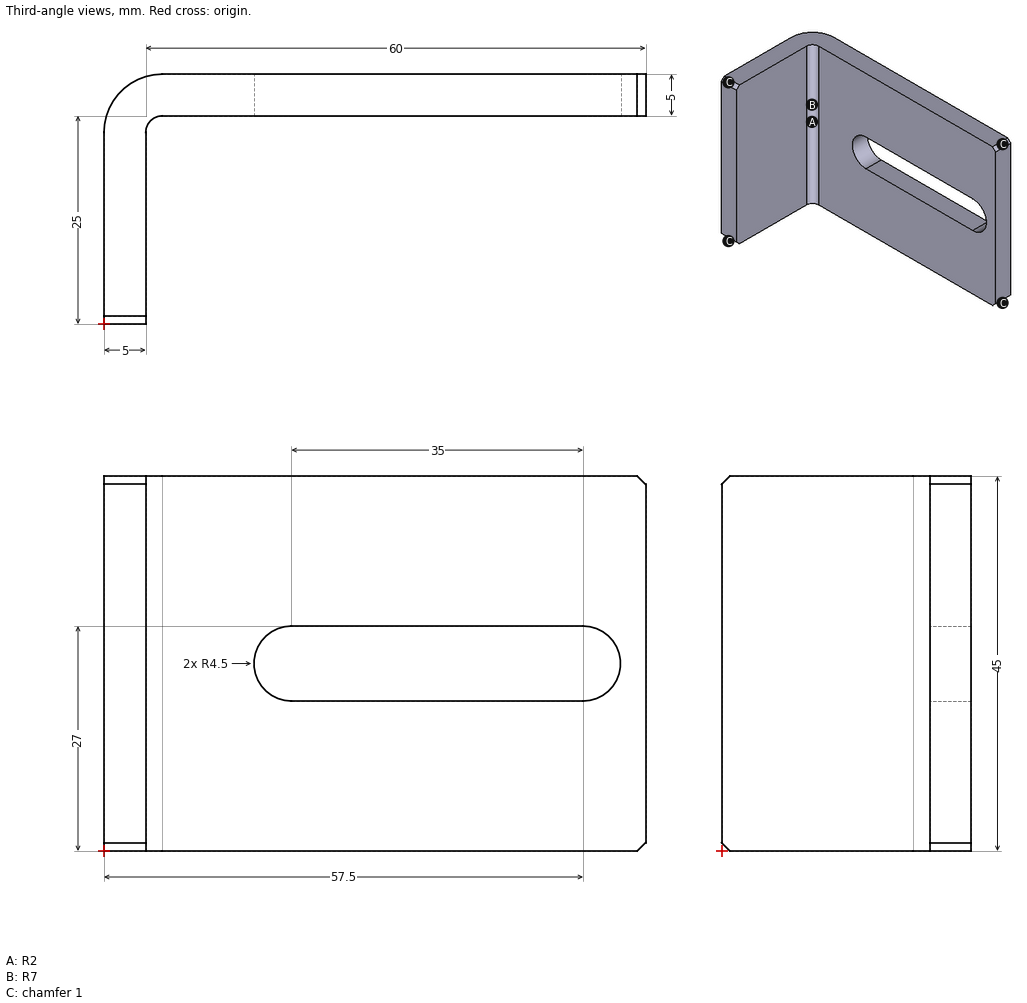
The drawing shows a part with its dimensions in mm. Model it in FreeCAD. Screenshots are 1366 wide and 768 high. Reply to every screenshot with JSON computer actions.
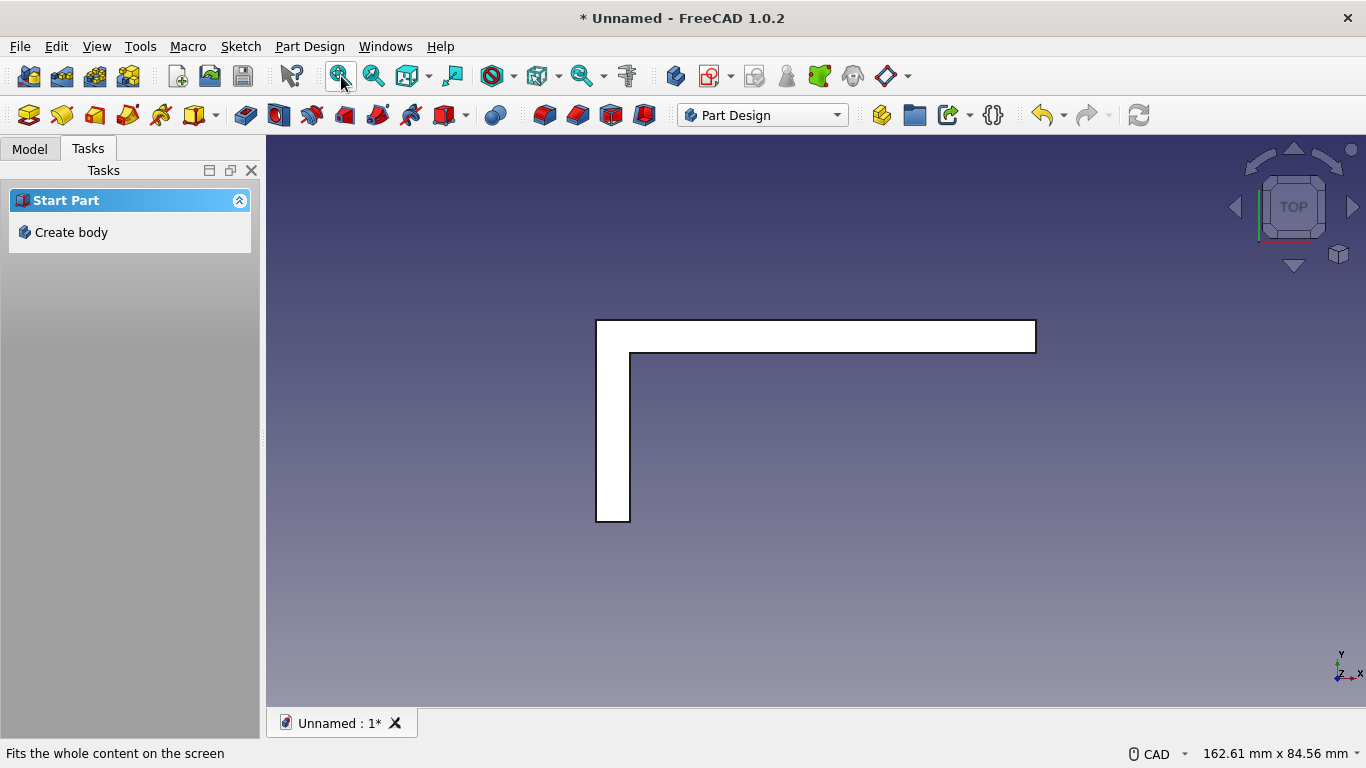
{"action": "key", "text": "1"}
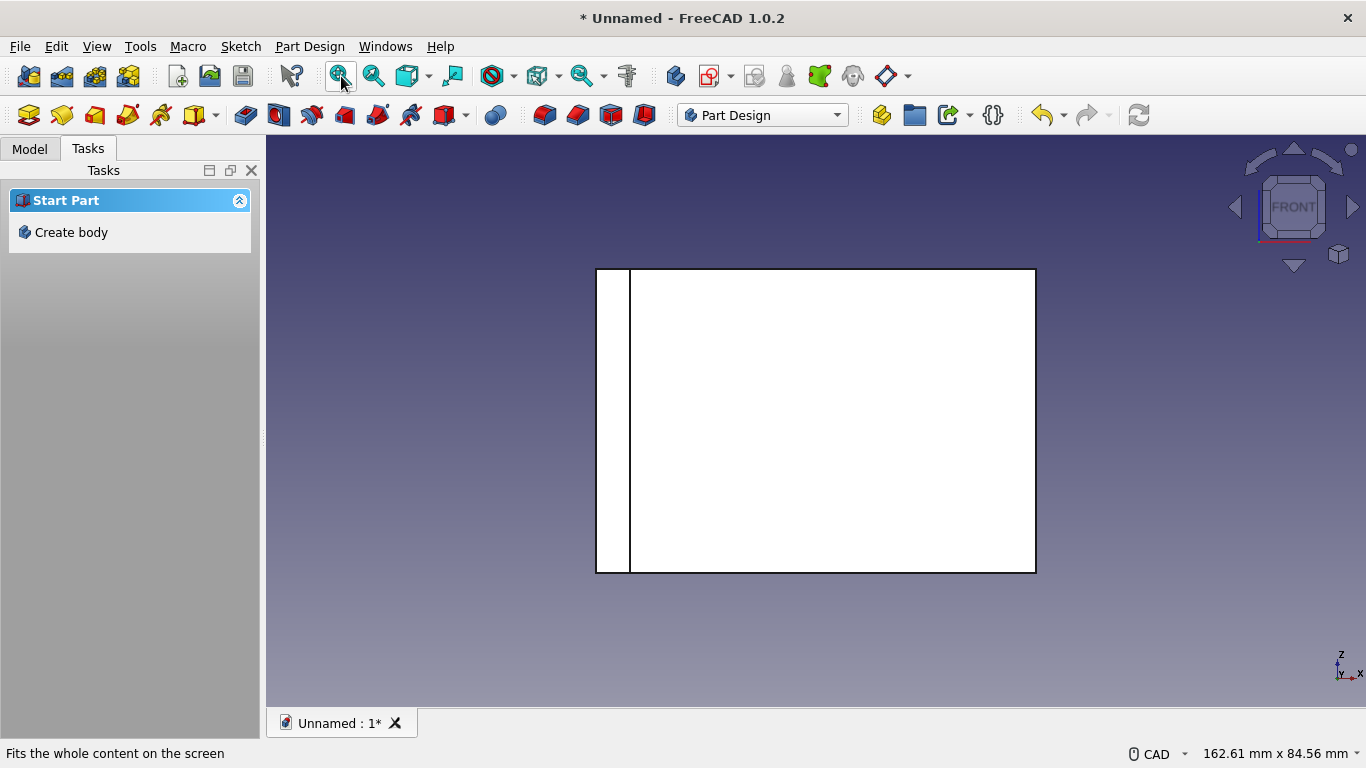
{"action": "key", "text": "3"}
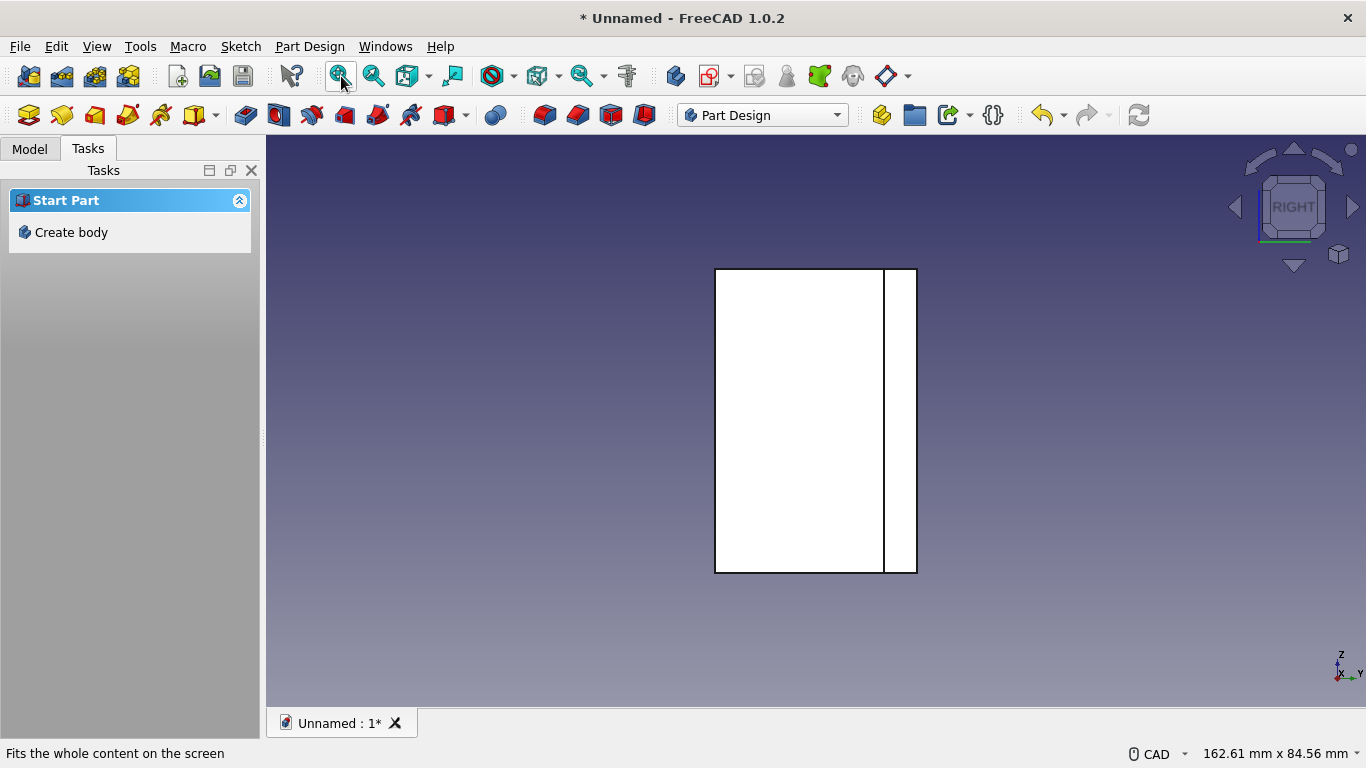
{"action": "key", "text": "5"}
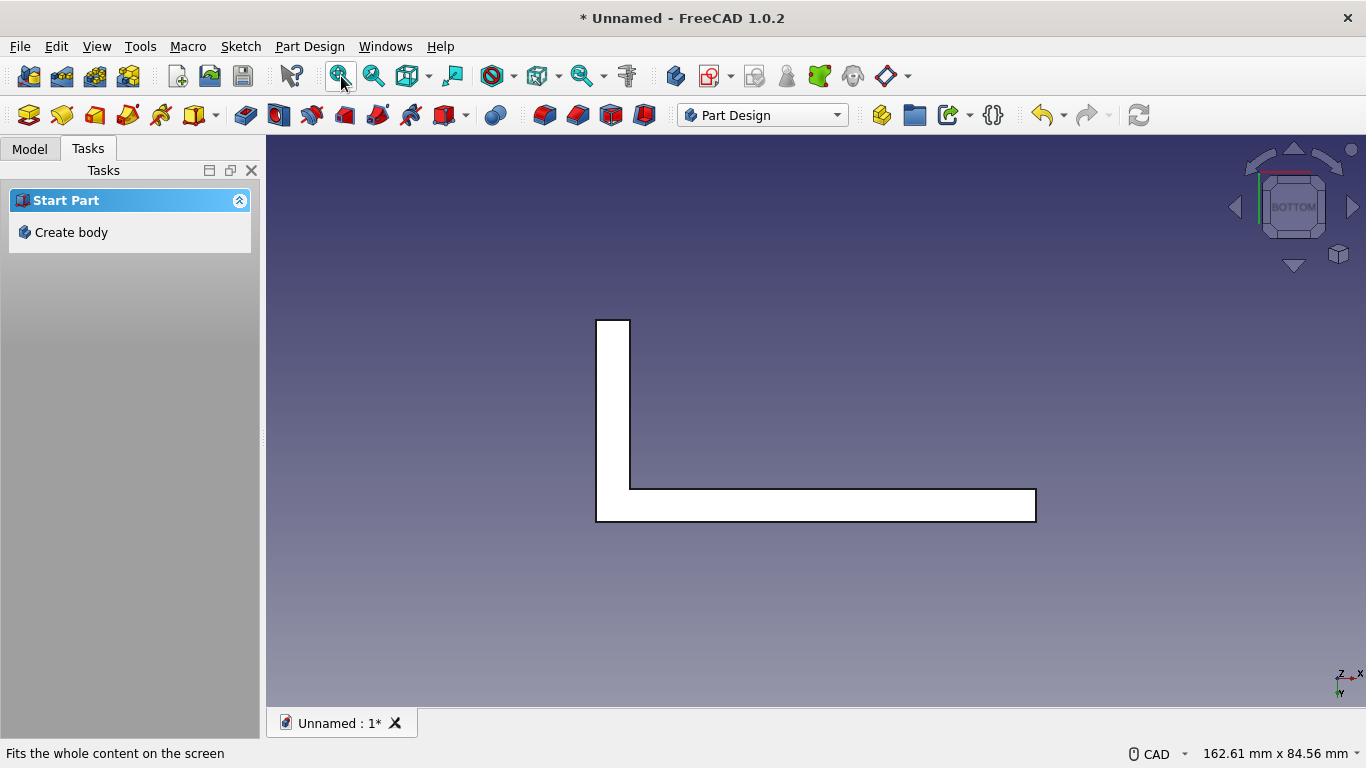
{"action": "left_click", "coordinate": [341, 76]}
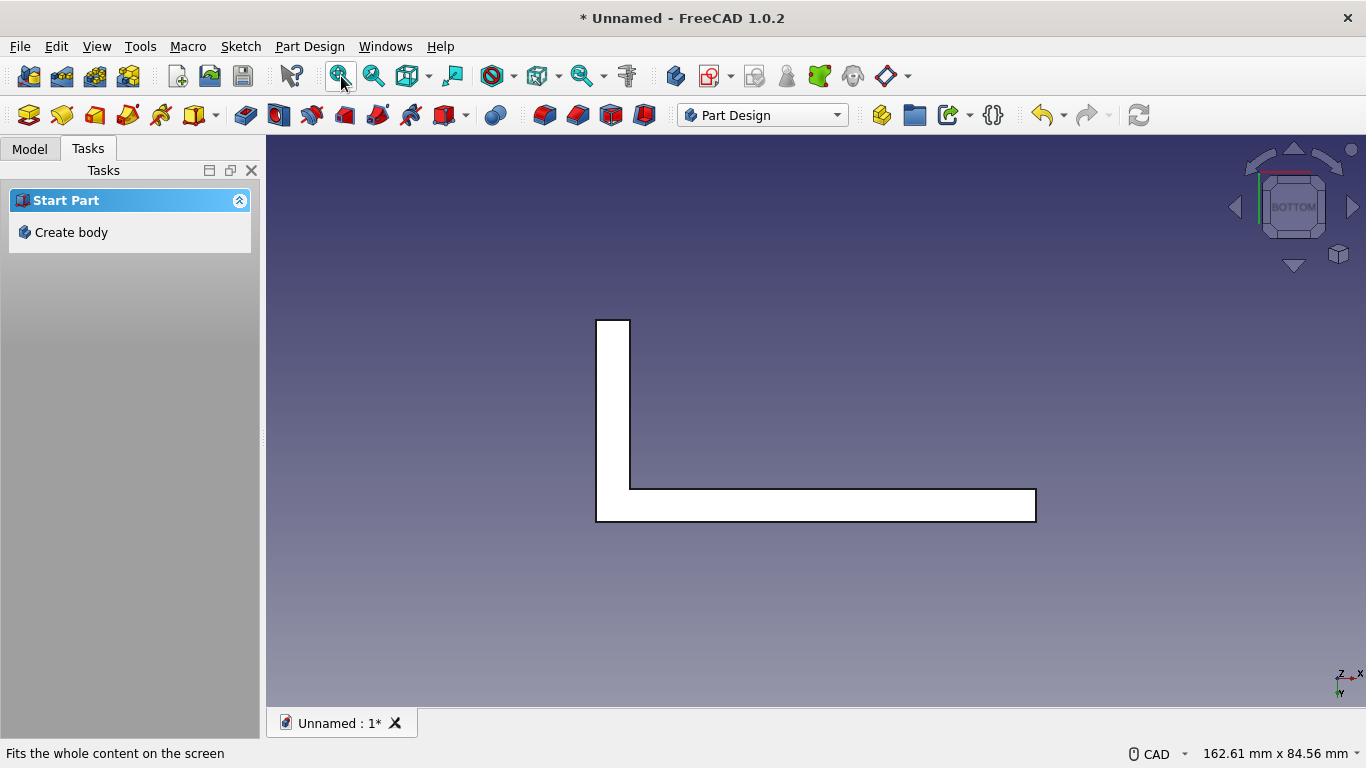
{"action": "key", "text": "4"}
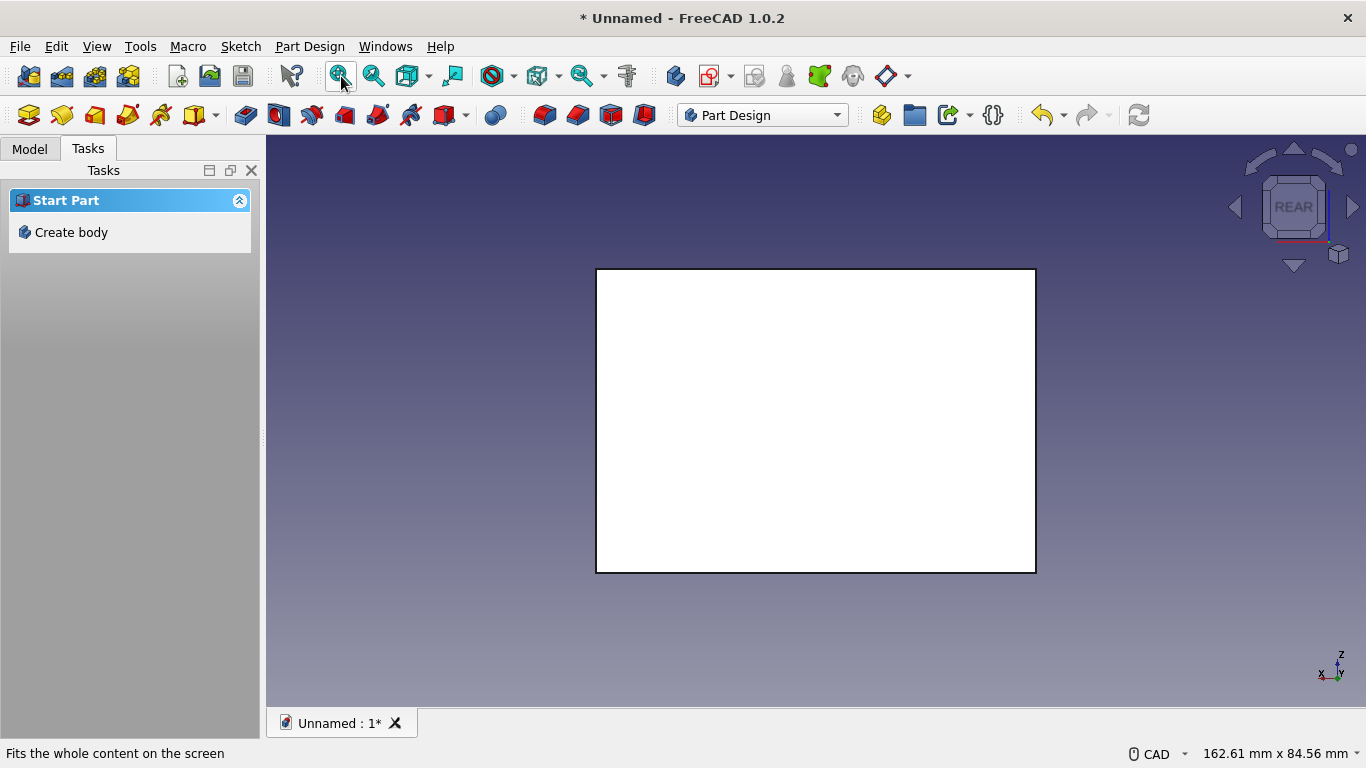
{"action": "key", "text": "6"}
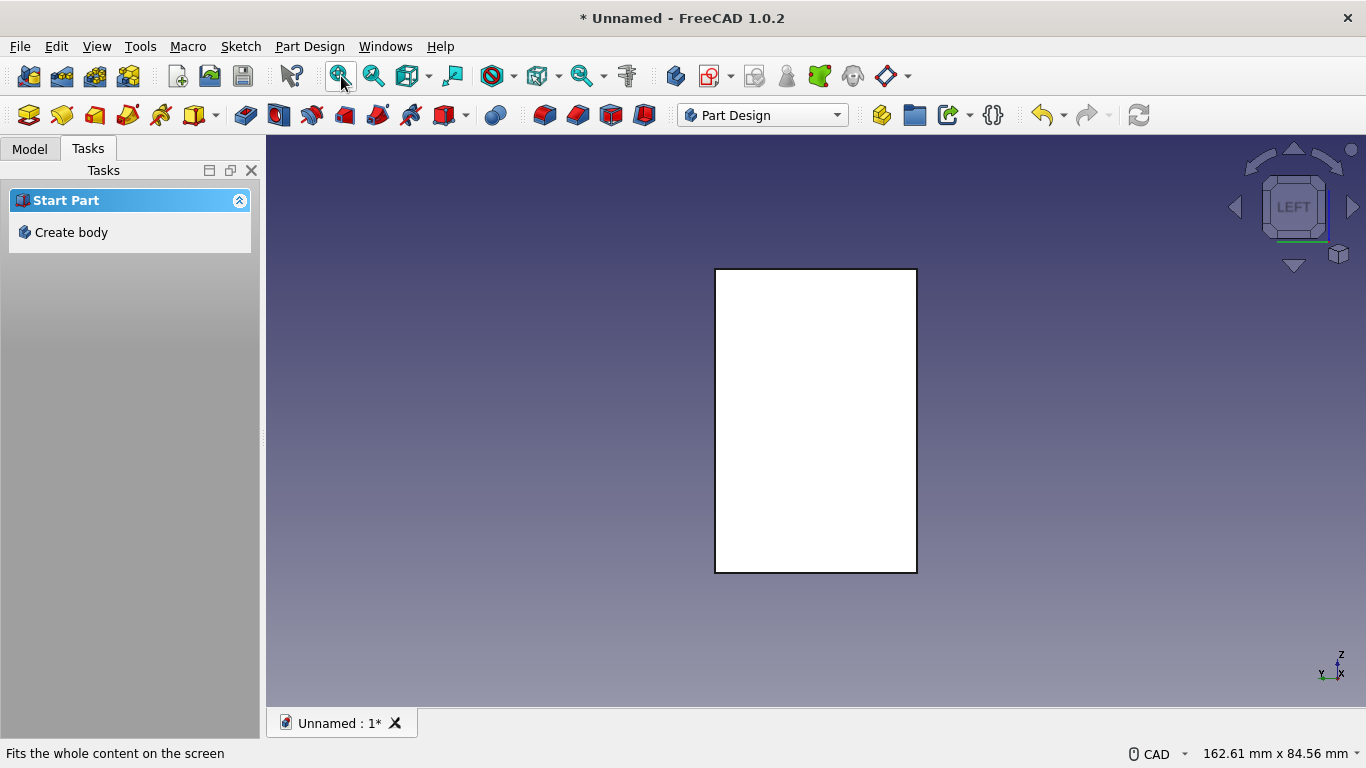
{"action": "key", "text": "v 3"}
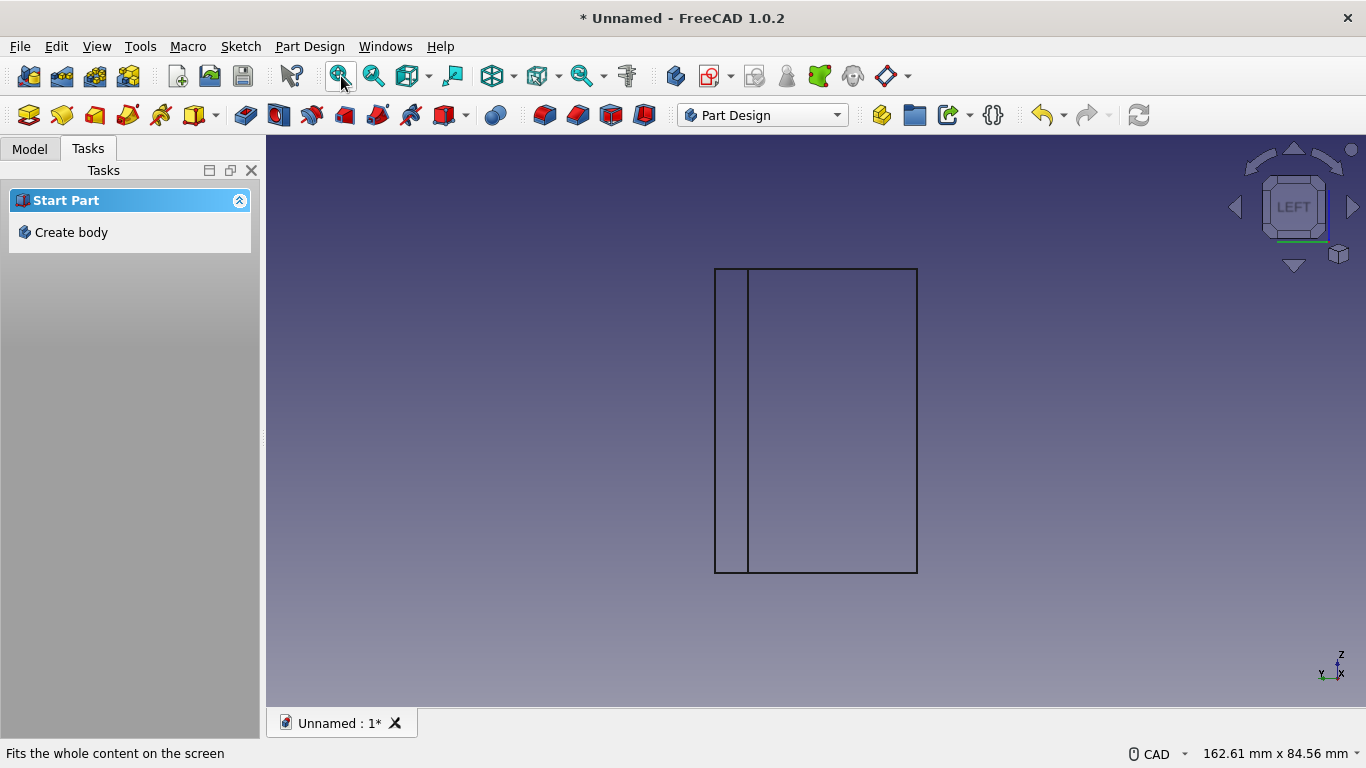
{"action": "key", "text": "0"}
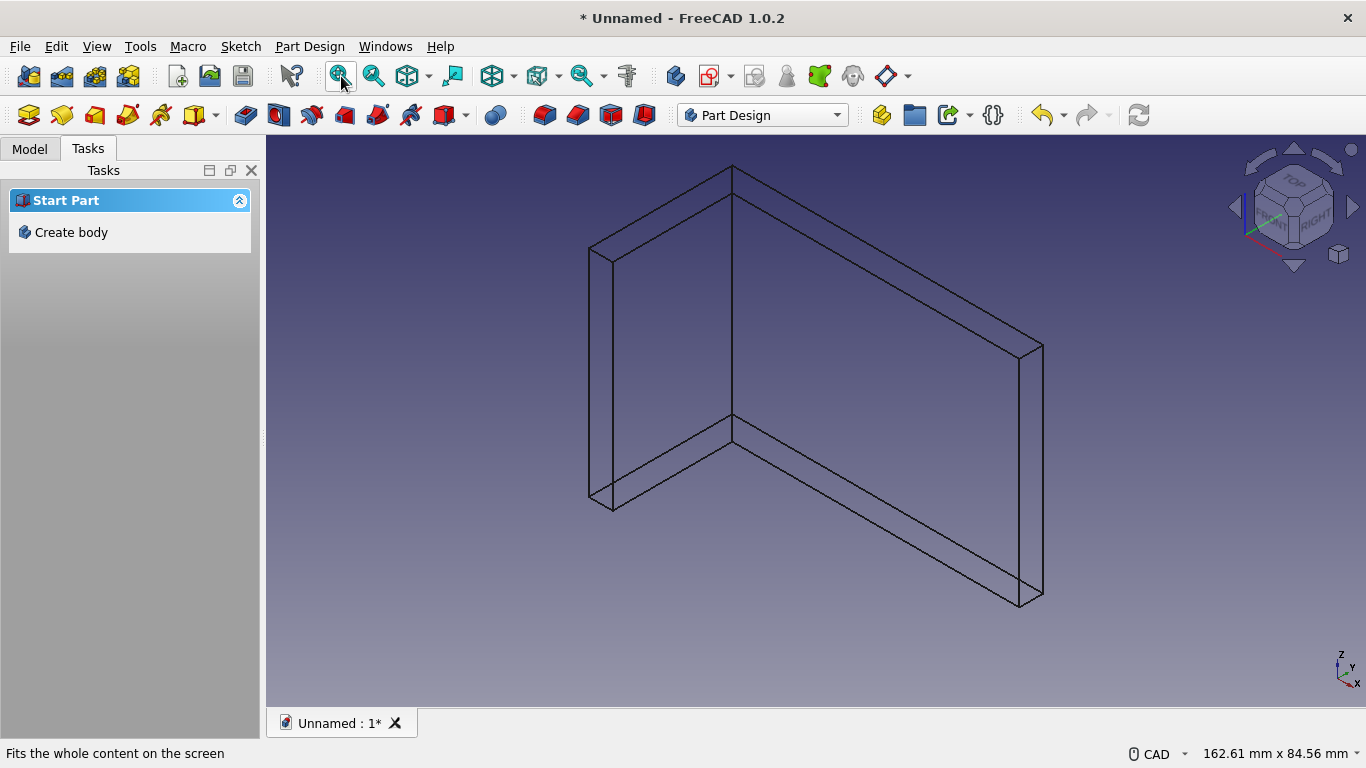
{"action": "left_click", "coordinate": [732, 316]}